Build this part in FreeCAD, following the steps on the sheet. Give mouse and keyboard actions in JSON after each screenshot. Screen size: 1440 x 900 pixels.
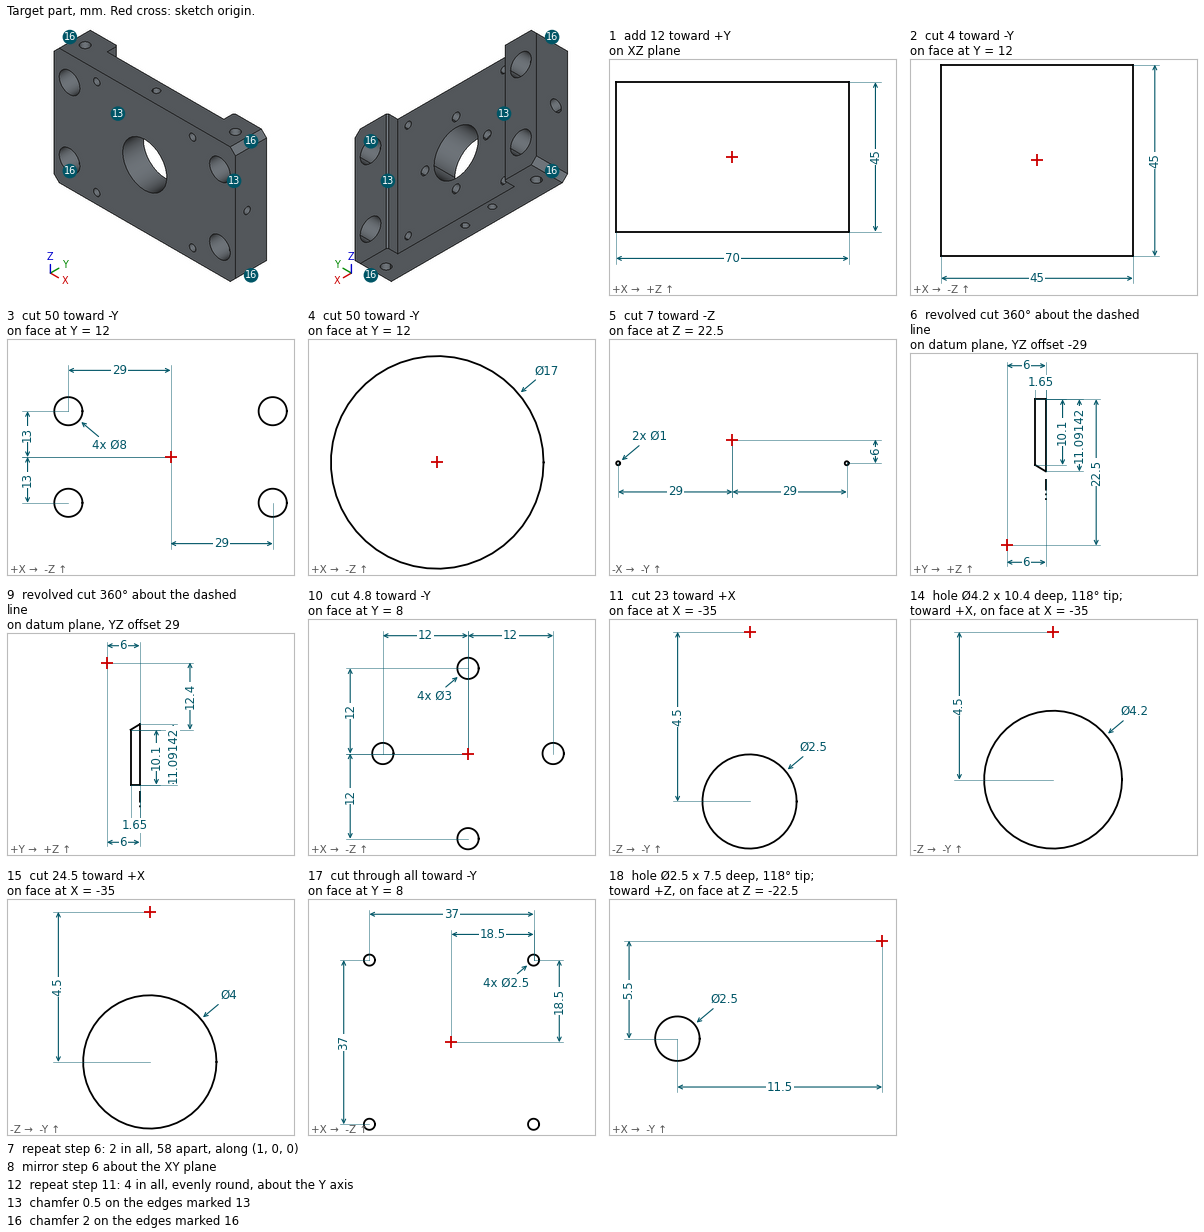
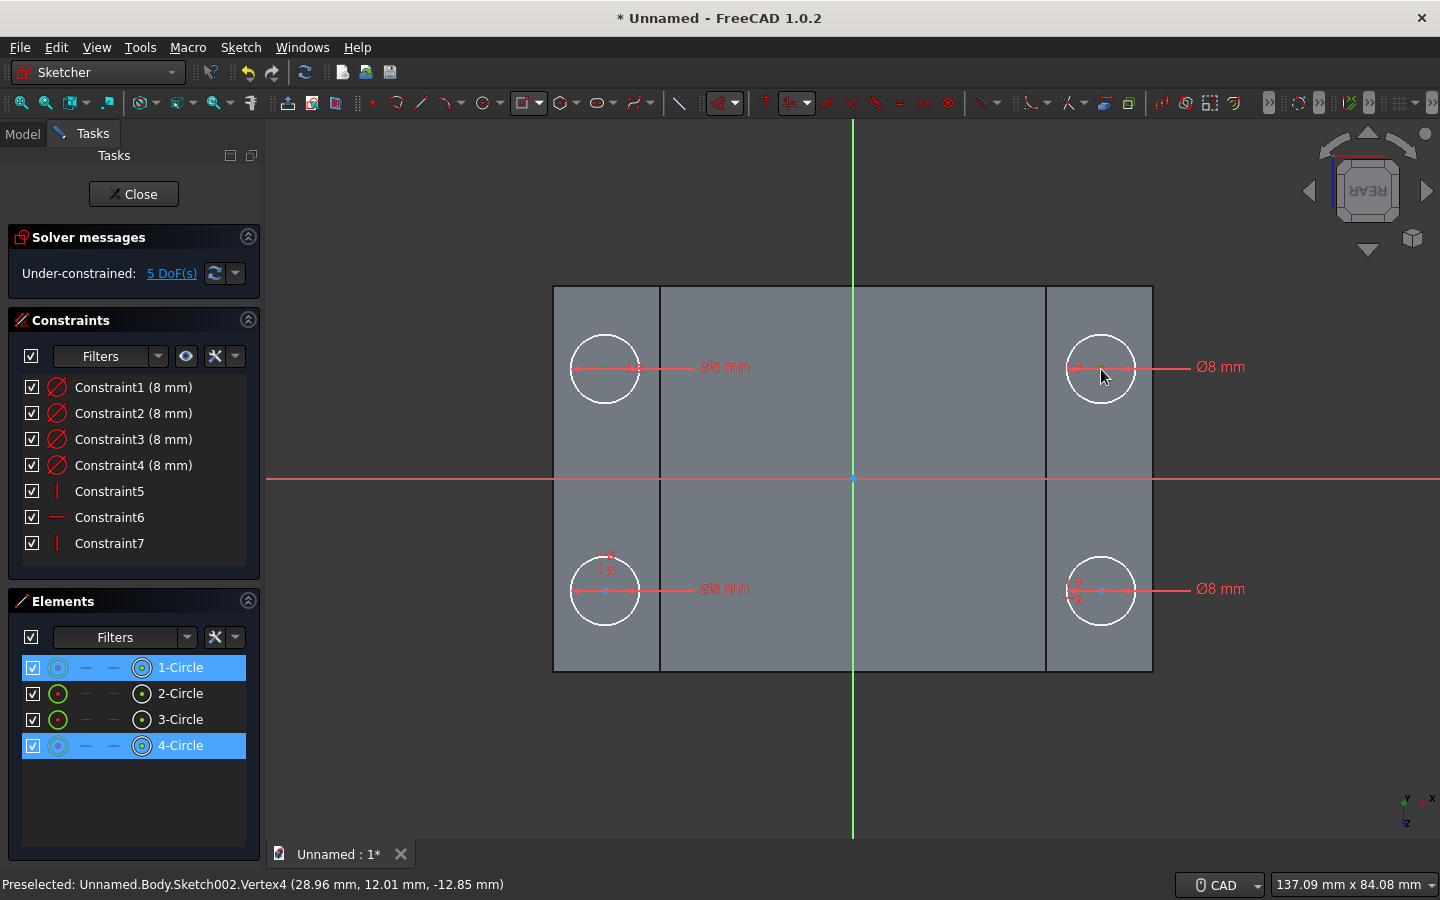
{"action": "key", "text": "h"}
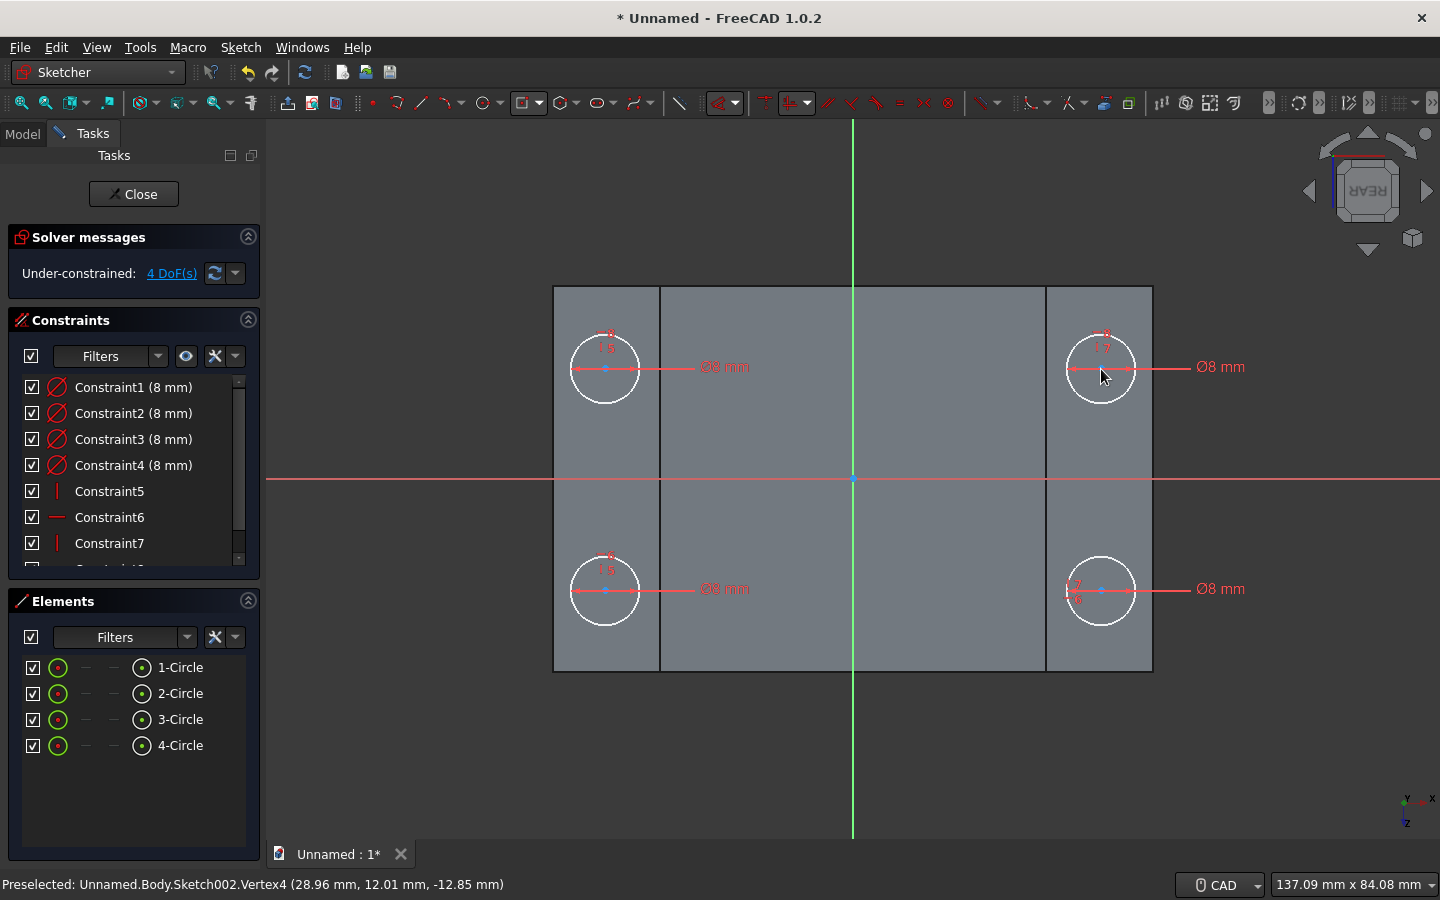
{"action": "left_click", "coordinate": [718, 104]}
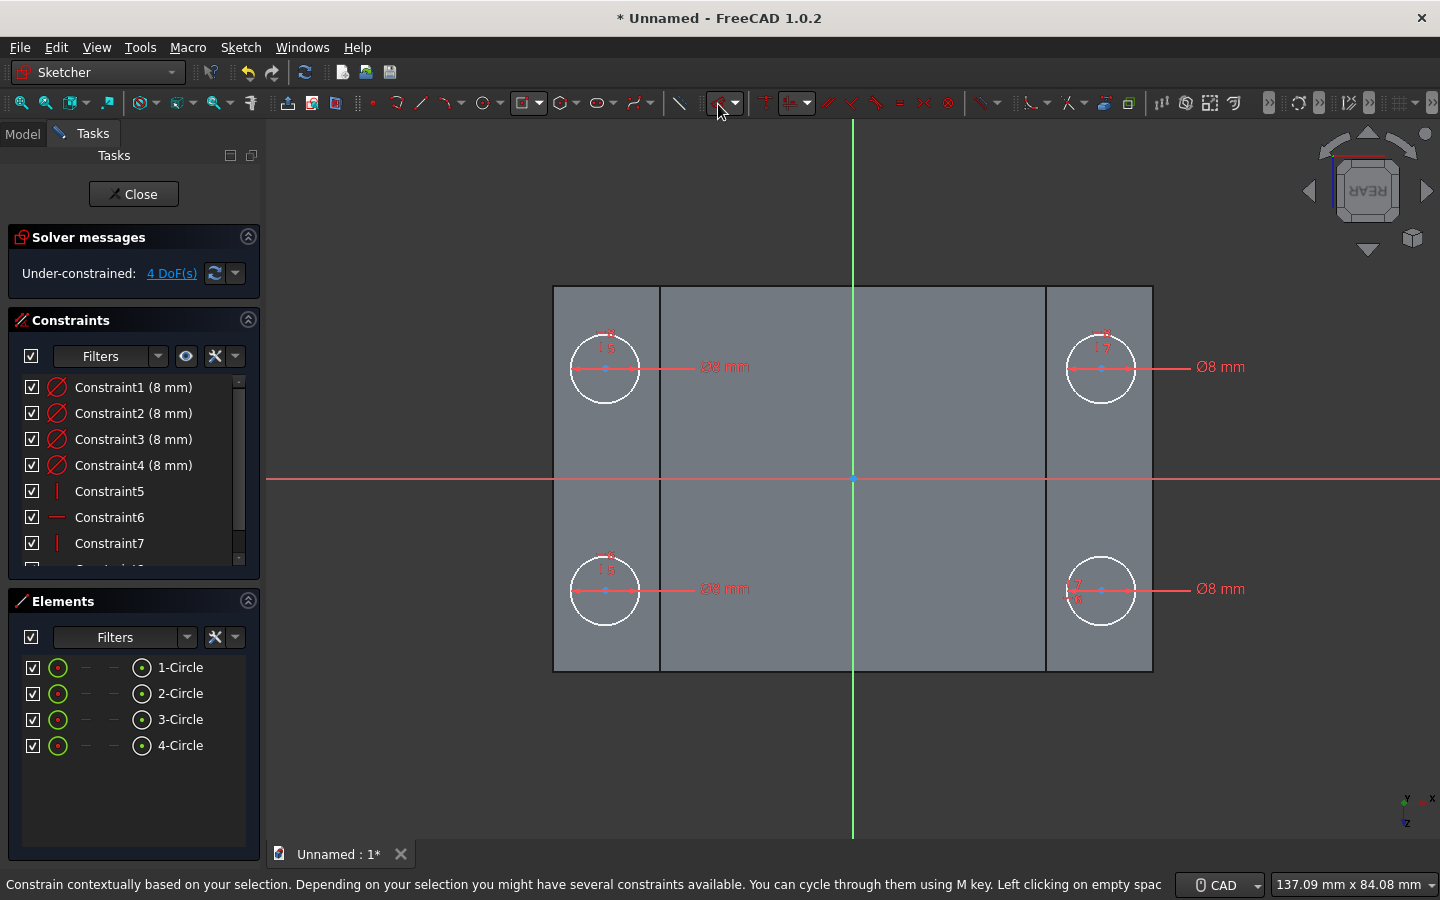
{"action": "left_click", "coordinate": [605, 369]}
{"action": "left_click", "coordinate": [729, 335]}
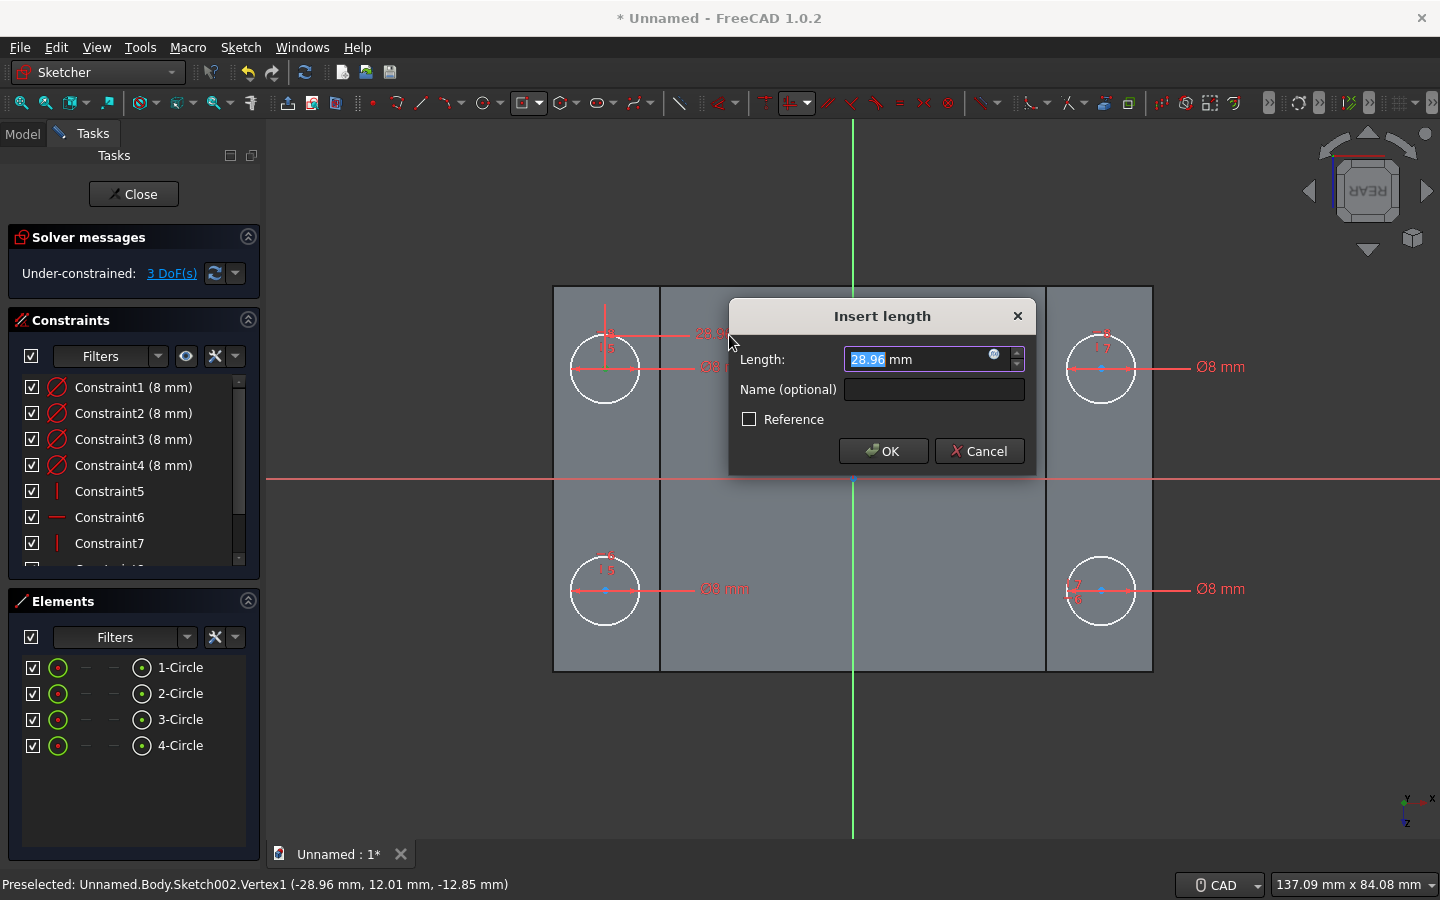
{"action": "type", "text": "29"}
{"action": "key", "text": "Return"}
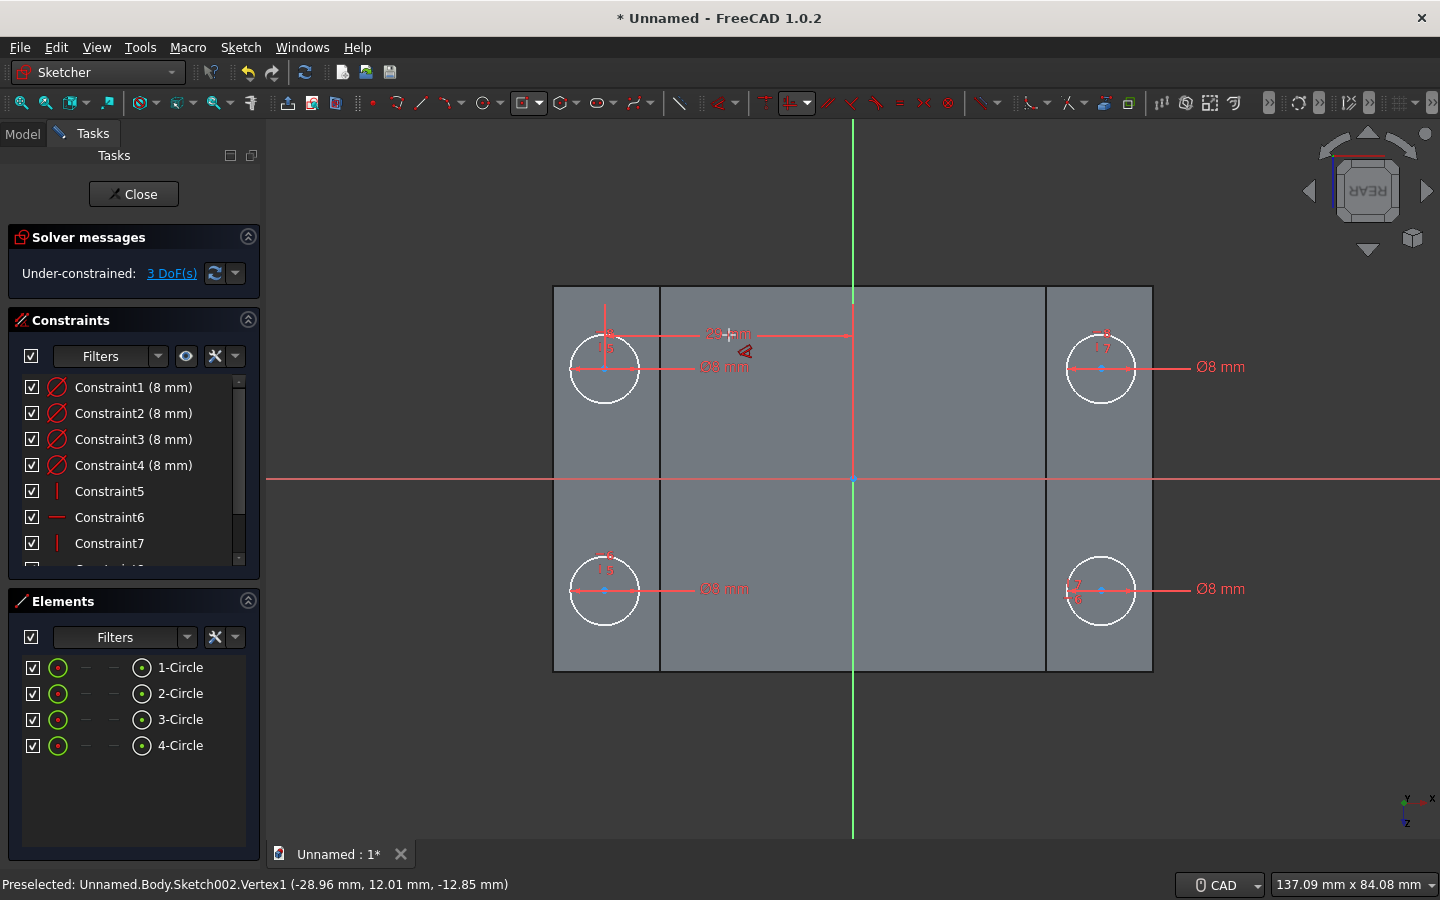
{"action": "left_click", "coordinate": [605, 369]}
{"action": "left_click", "coordinate": [571, 424]}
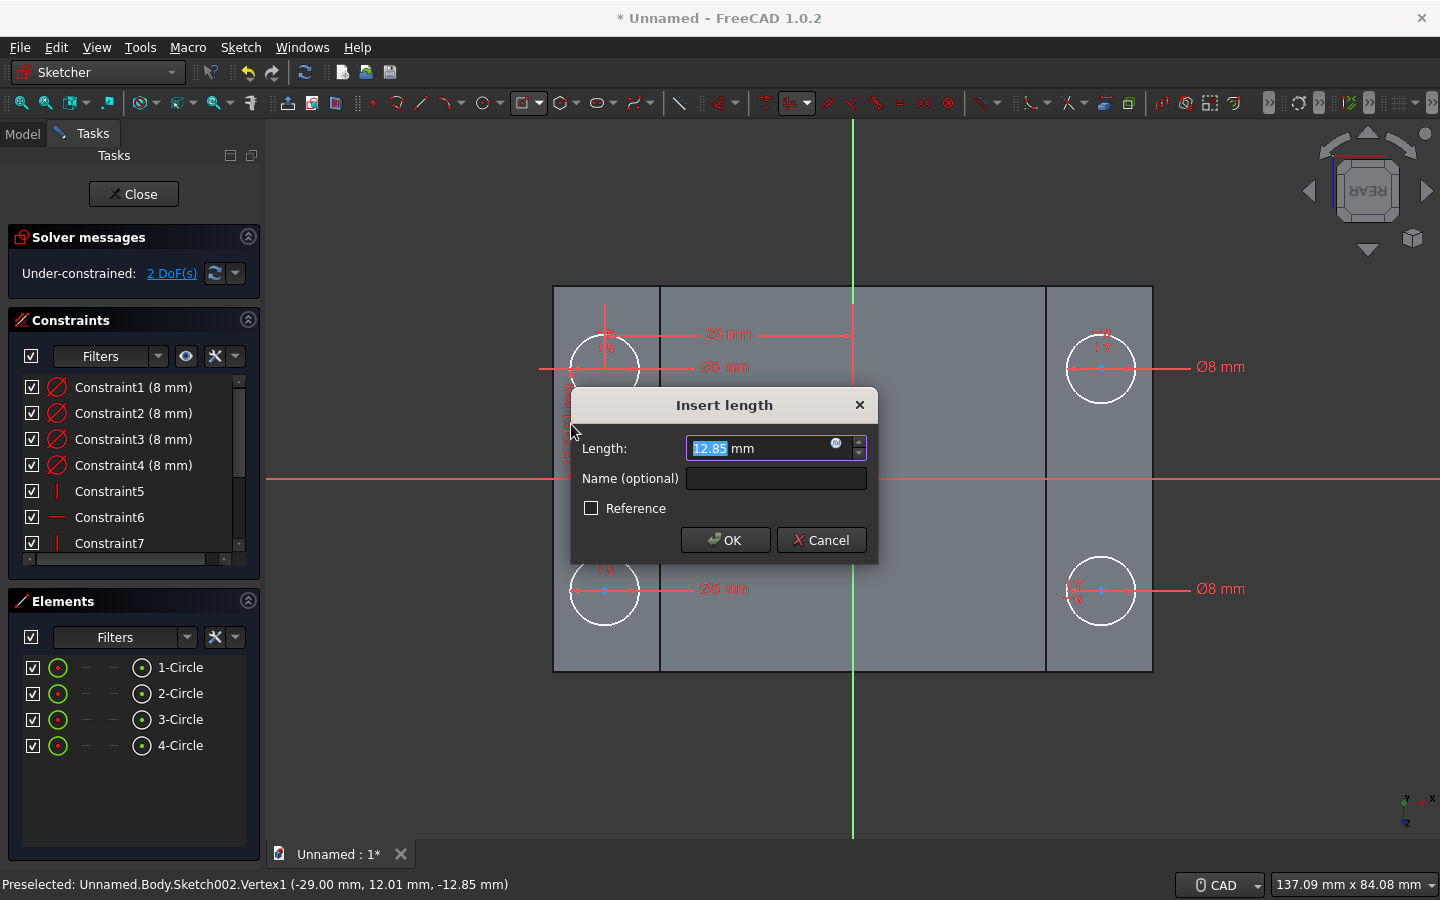
{"action": "type", "text": "13"}
{"action": "key", "text": "Return"}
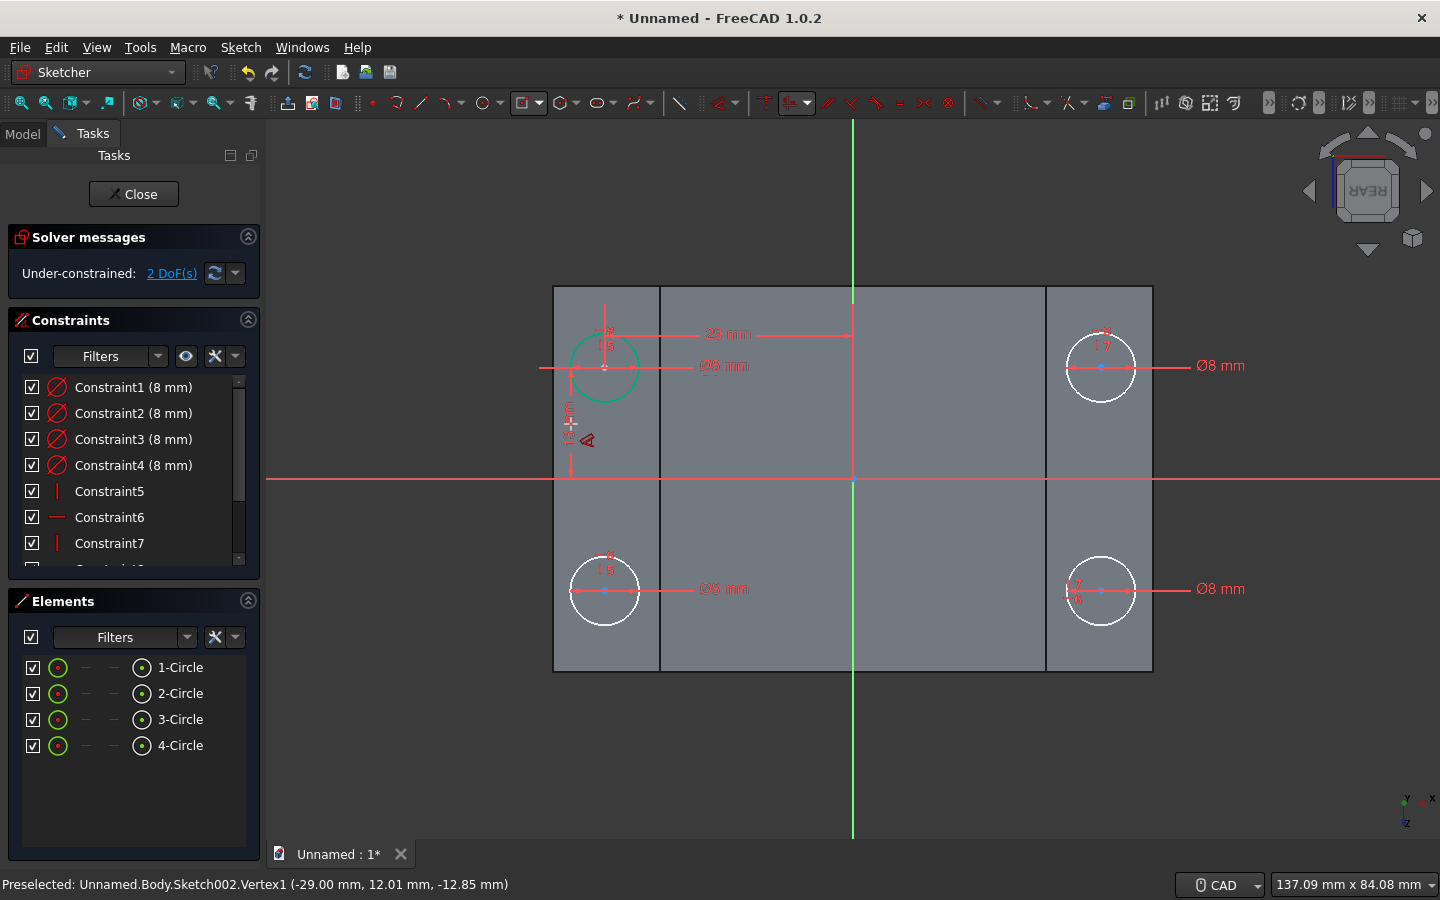
{"action": "left_click", "coordinate": [605, 591]}
{"action": "left_click", "coordinate": [571, 535]}